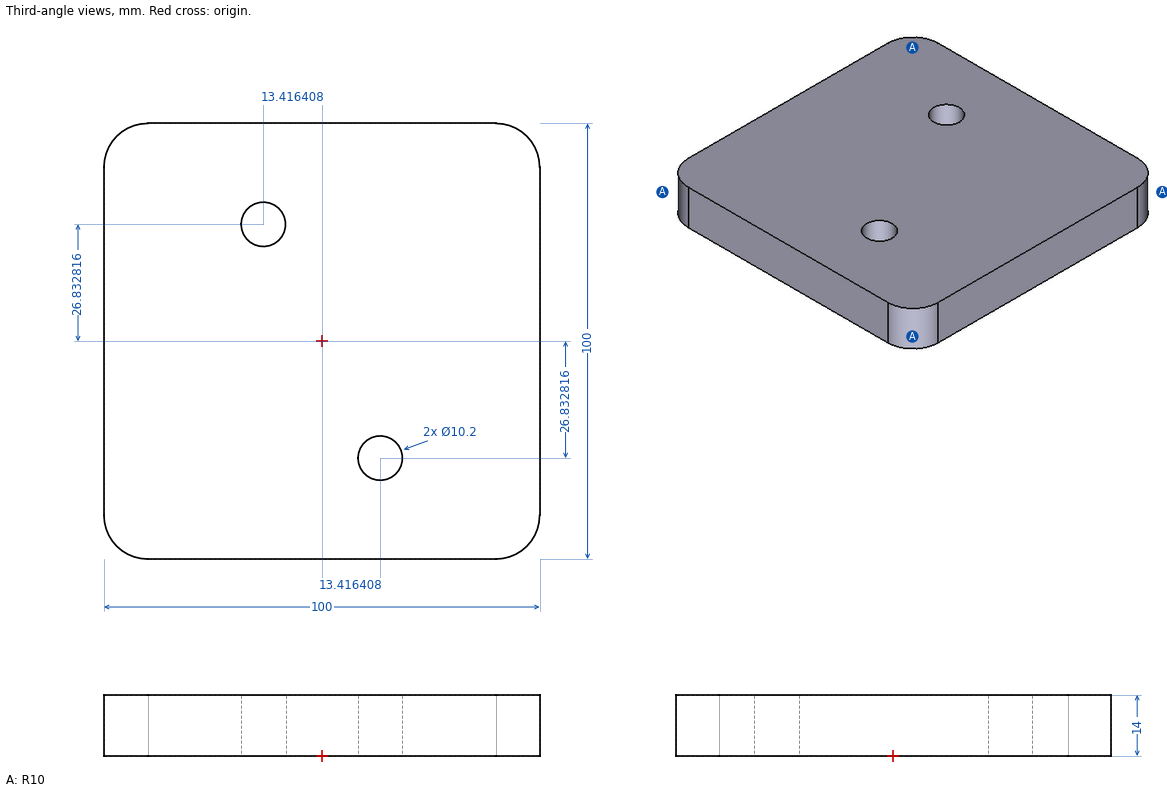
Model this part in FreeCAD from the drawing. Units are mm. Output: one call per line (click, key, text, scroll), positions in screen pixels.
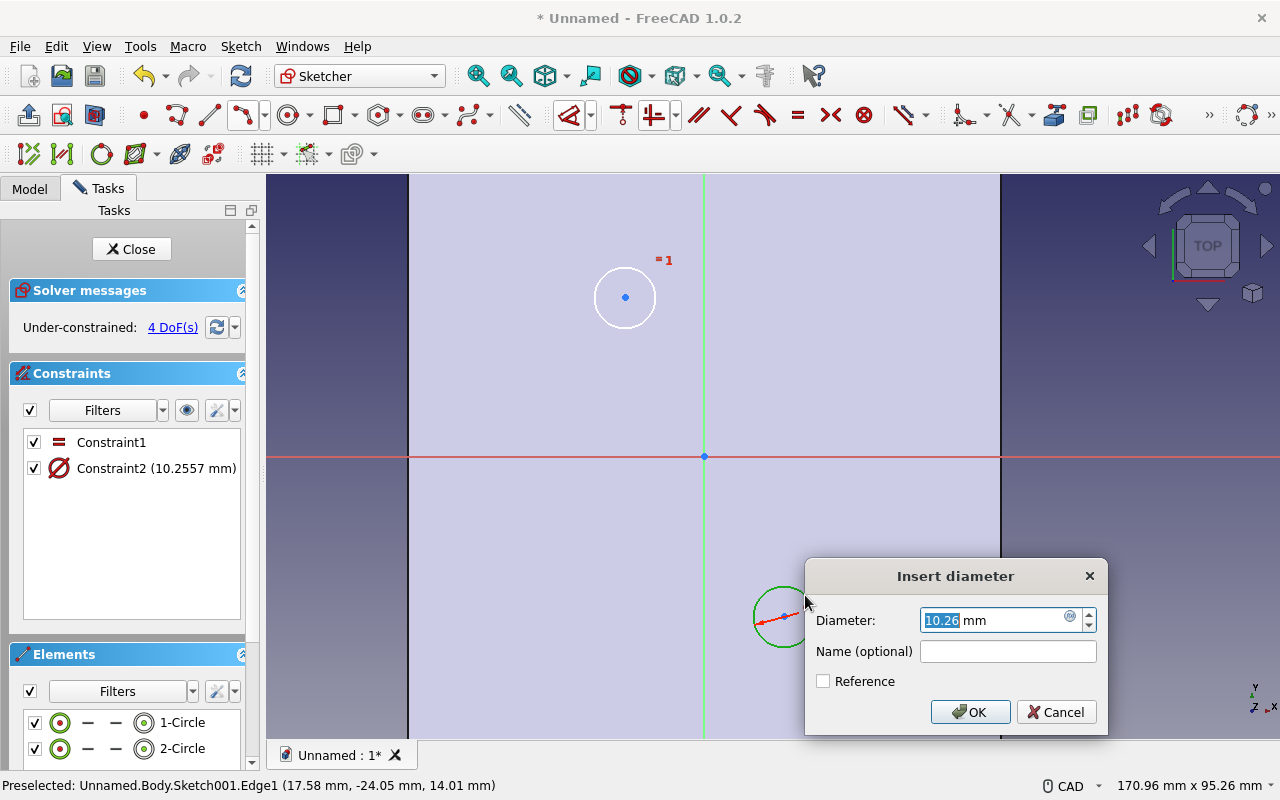
text(10.2)
key(Return)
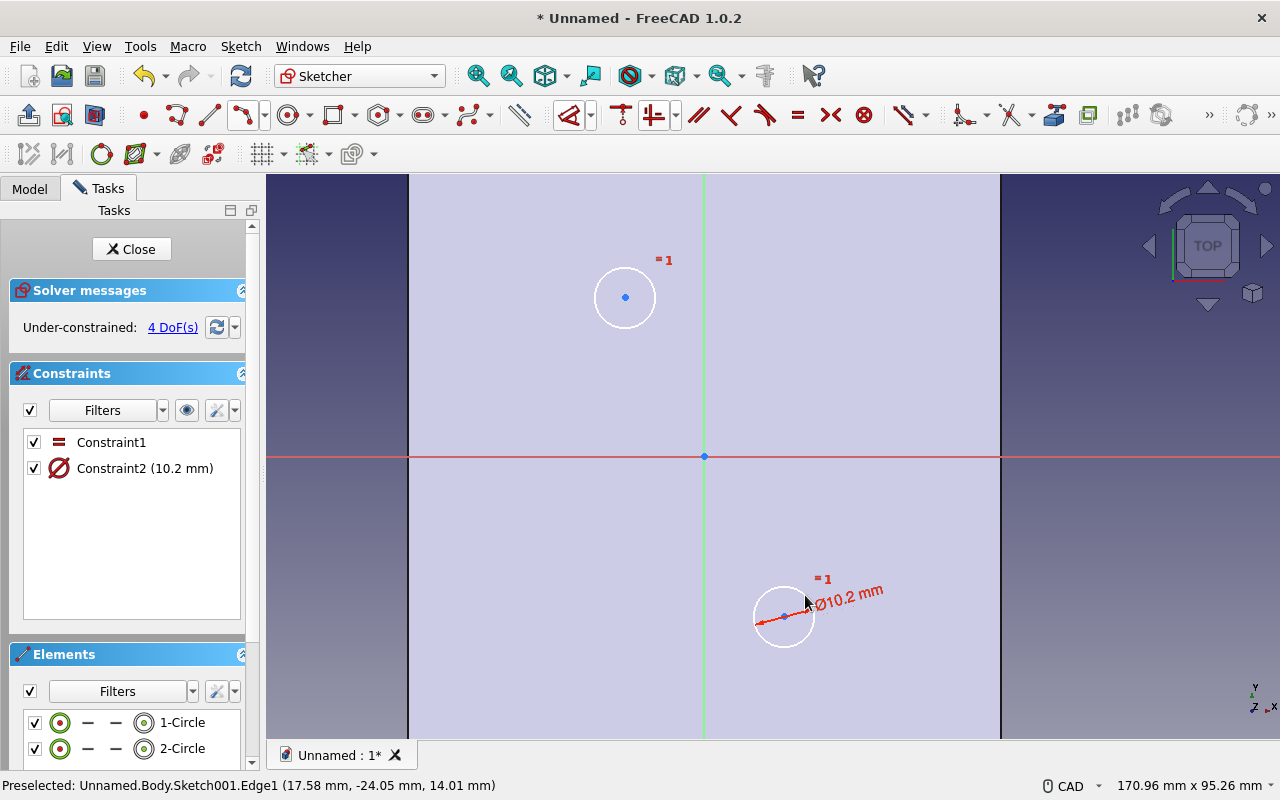
click(784, 617)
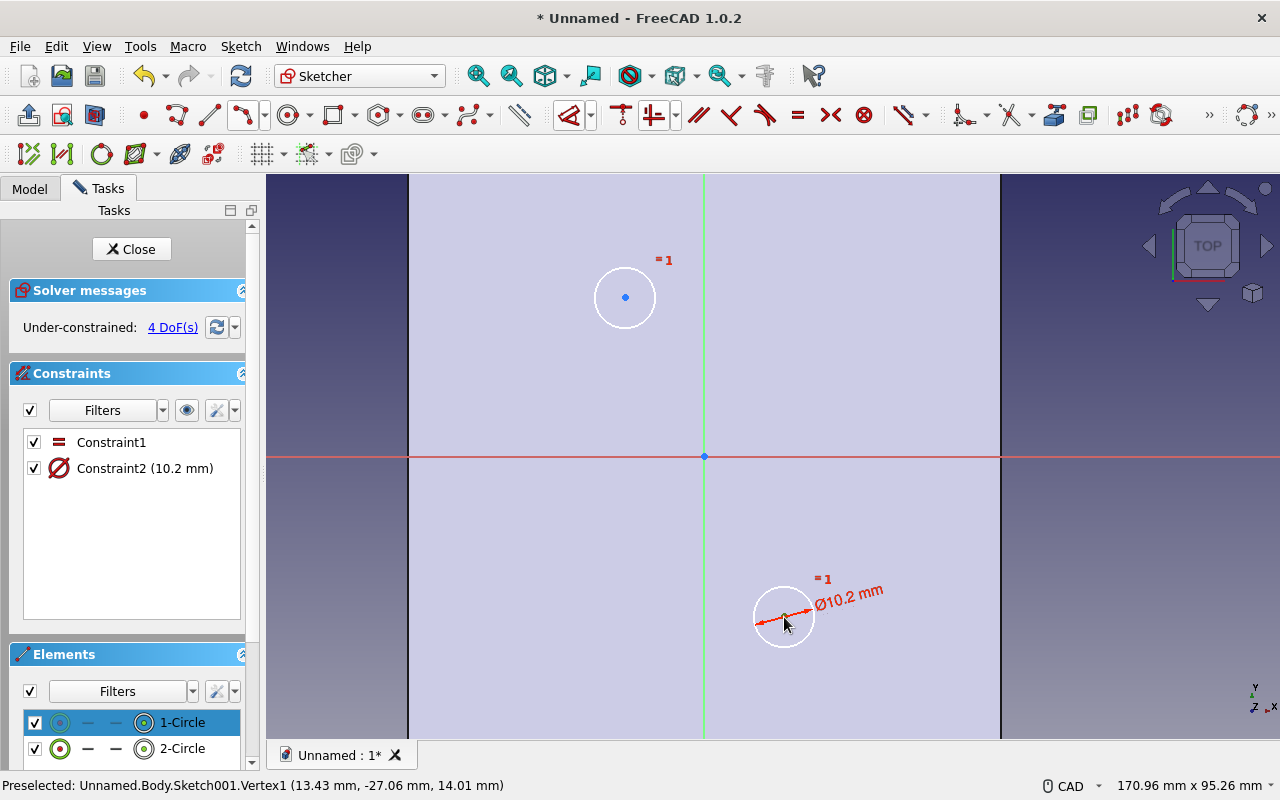
key(l)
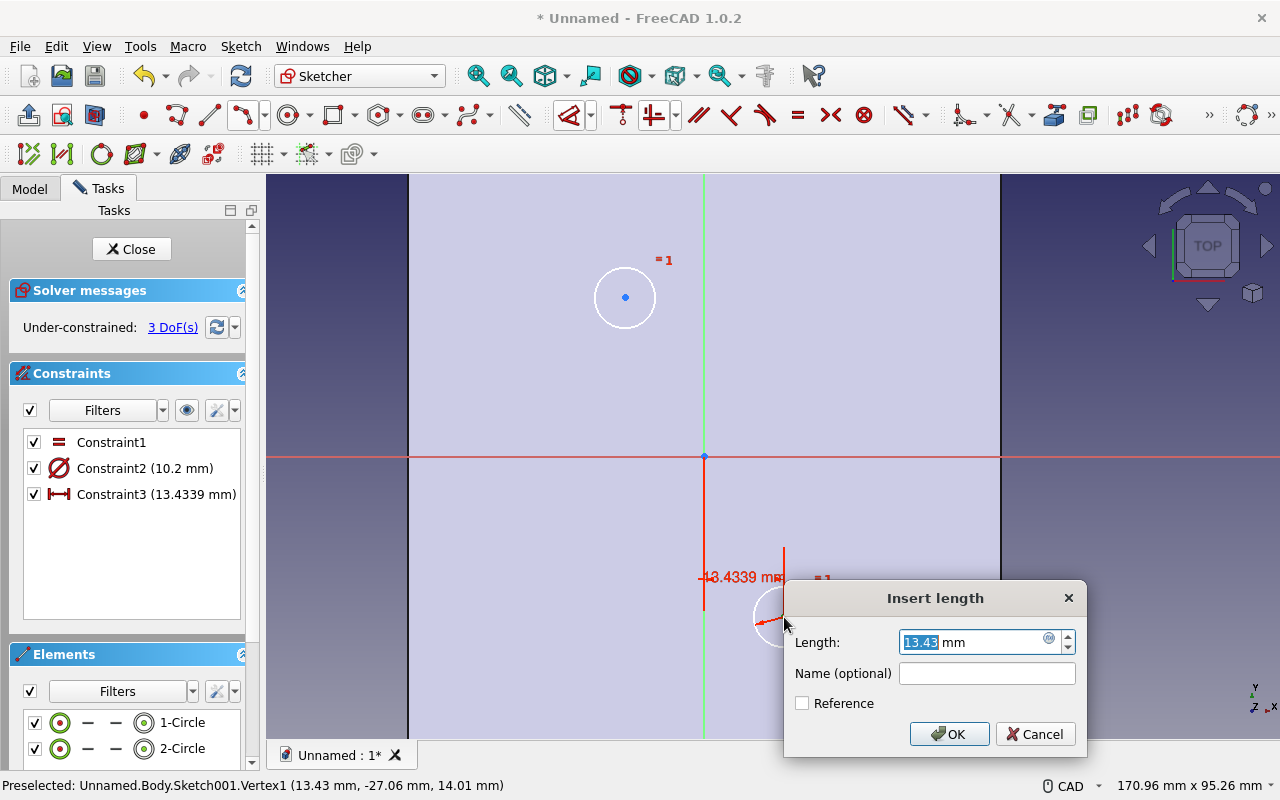
text(13.416408)
key(Return)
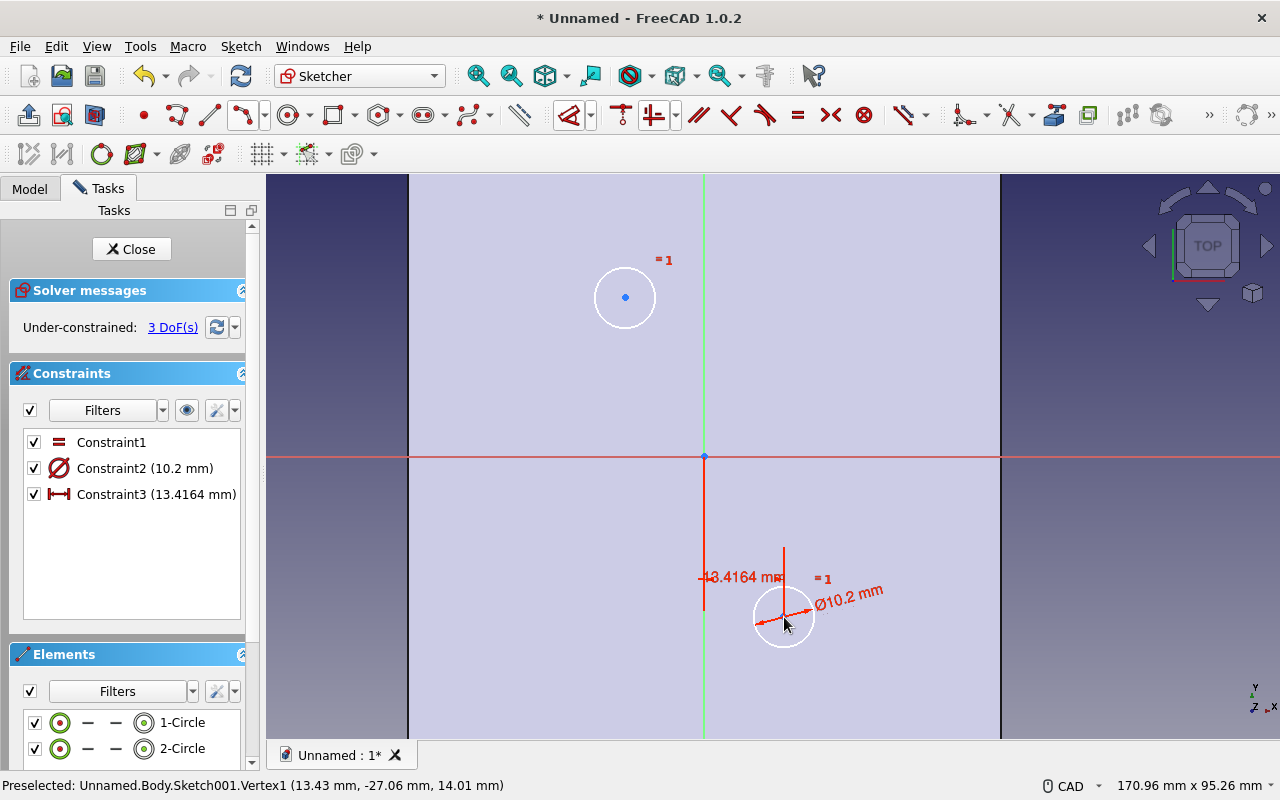
click(784, 617)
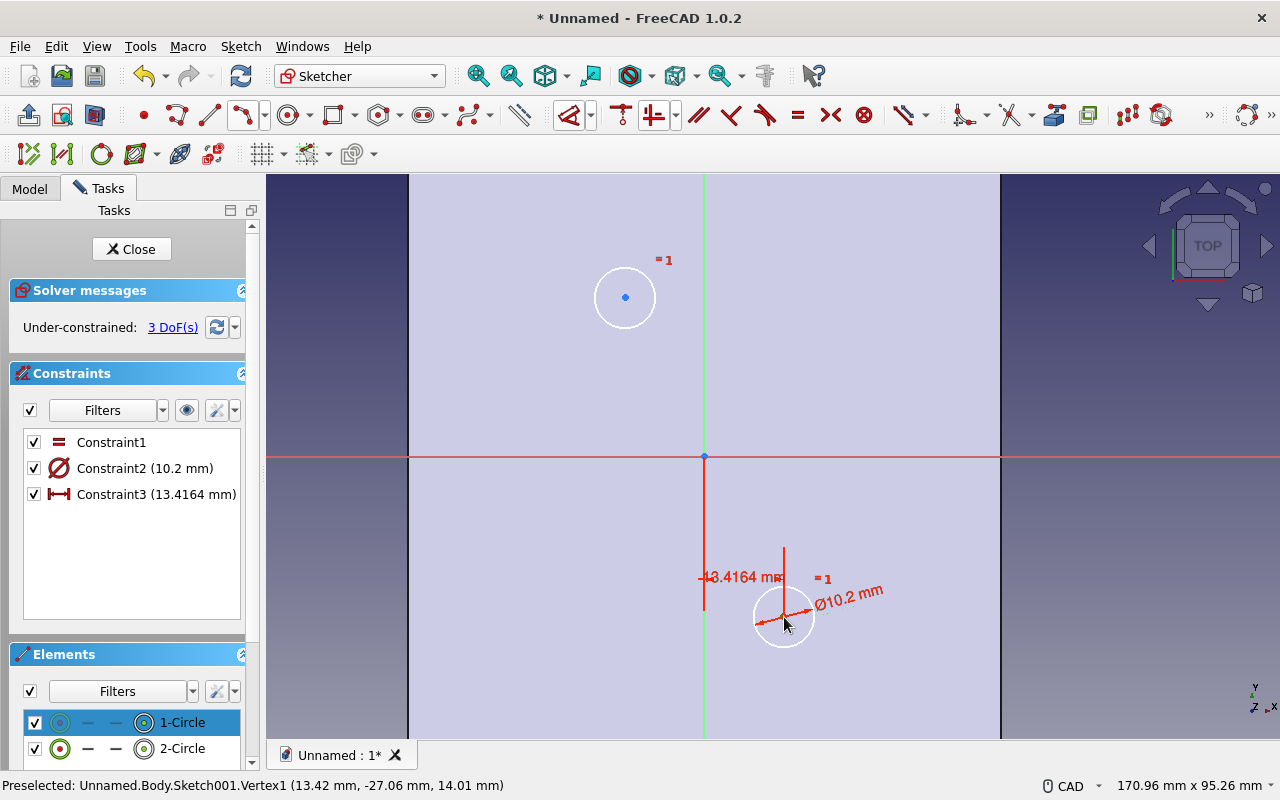
key(i)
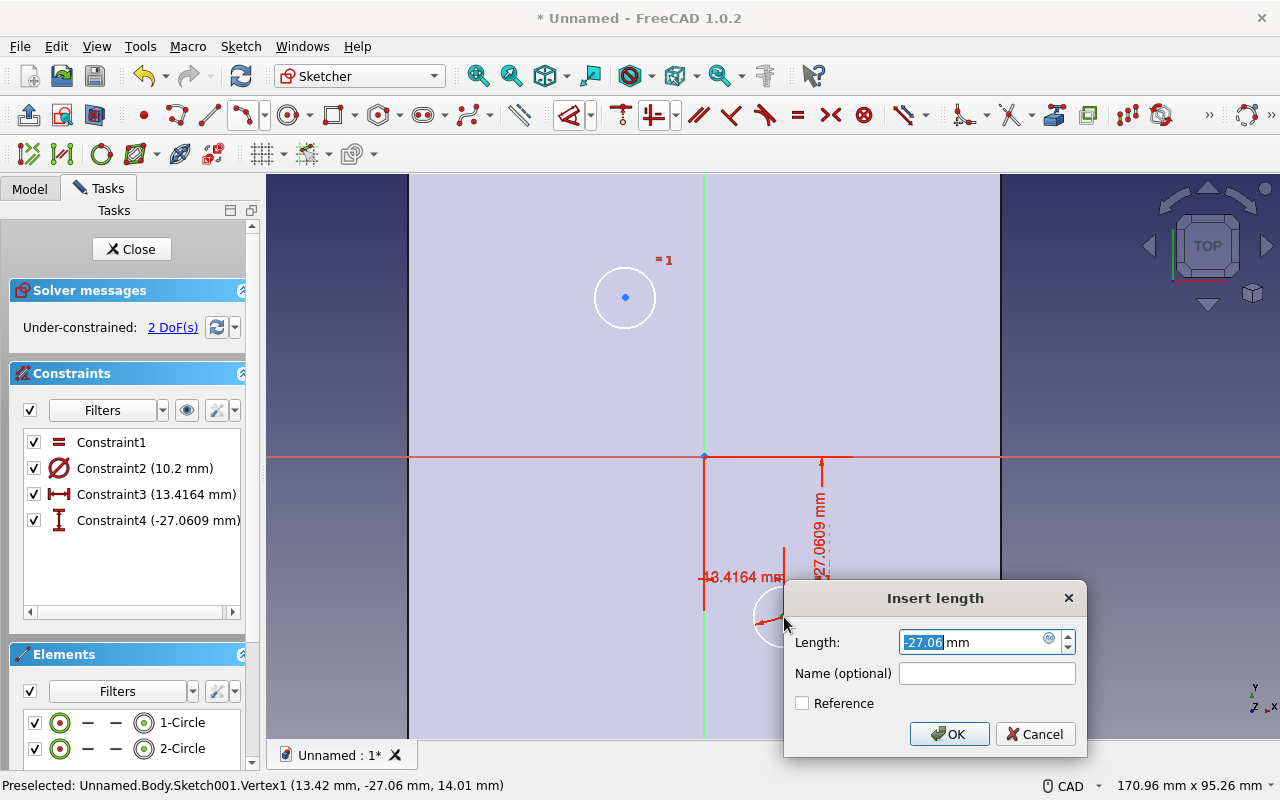
text(-26.832816)
key(Return)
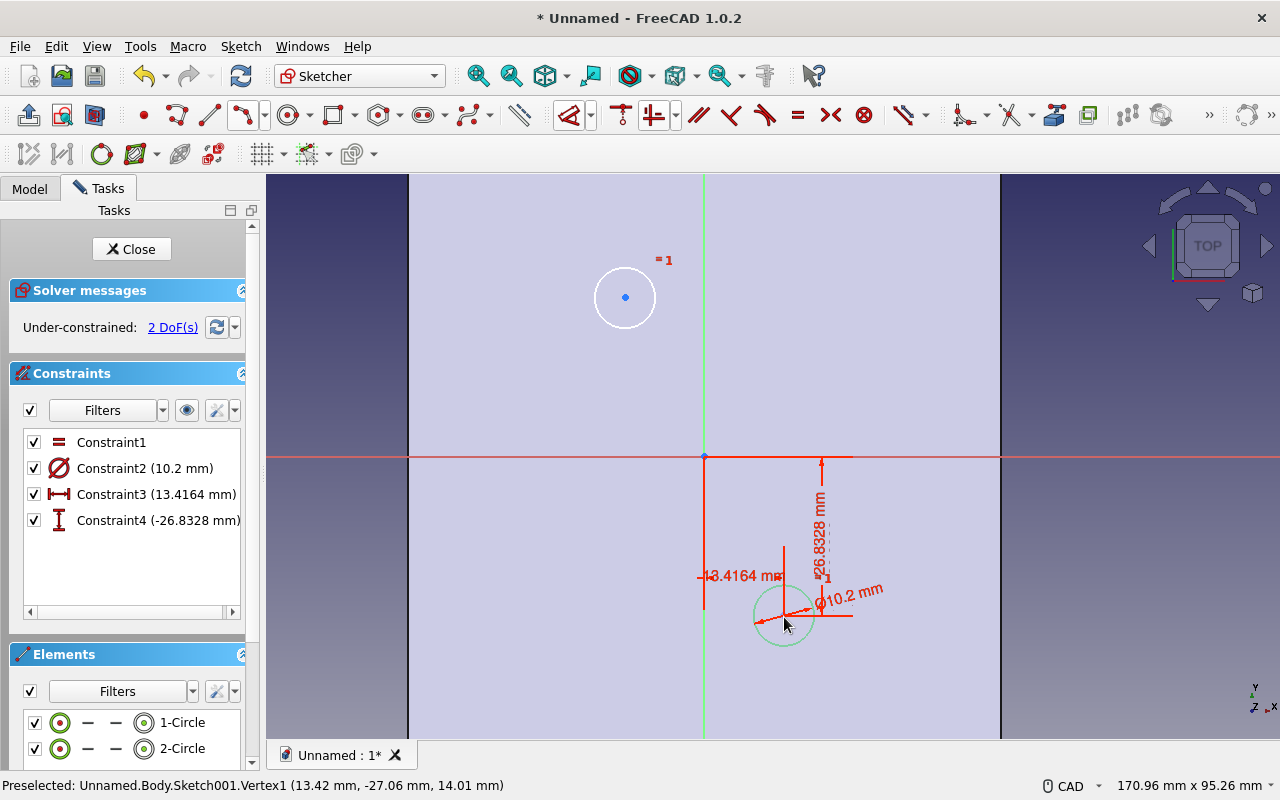
click(625, 298)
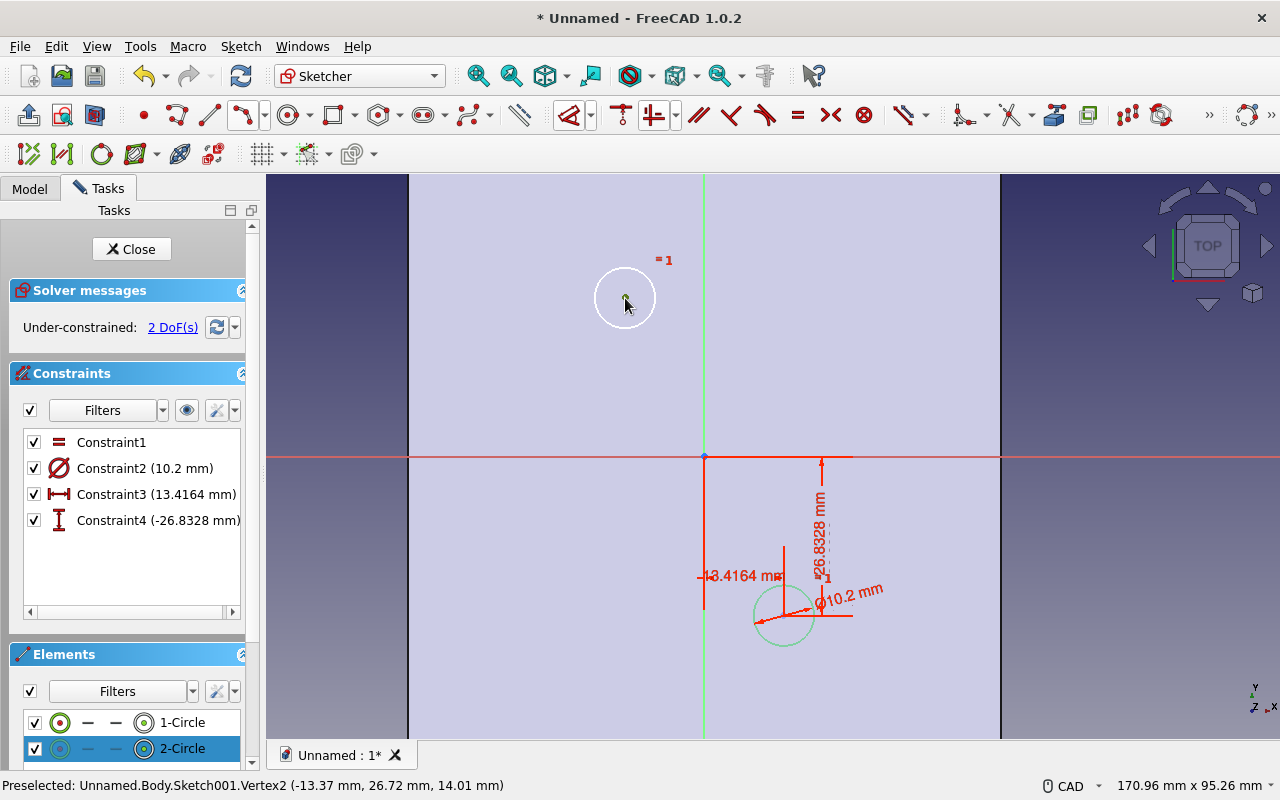
key(l)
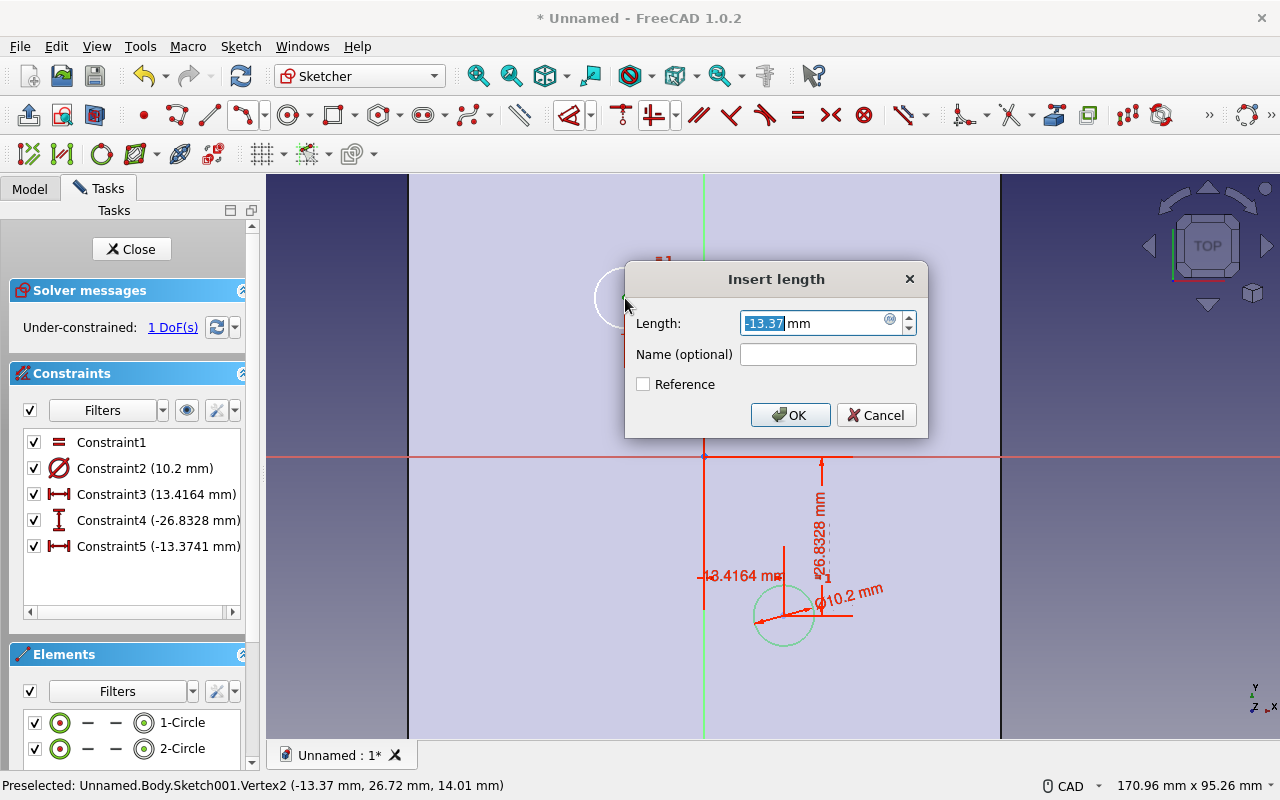
text(-13.416408)
key(Return)